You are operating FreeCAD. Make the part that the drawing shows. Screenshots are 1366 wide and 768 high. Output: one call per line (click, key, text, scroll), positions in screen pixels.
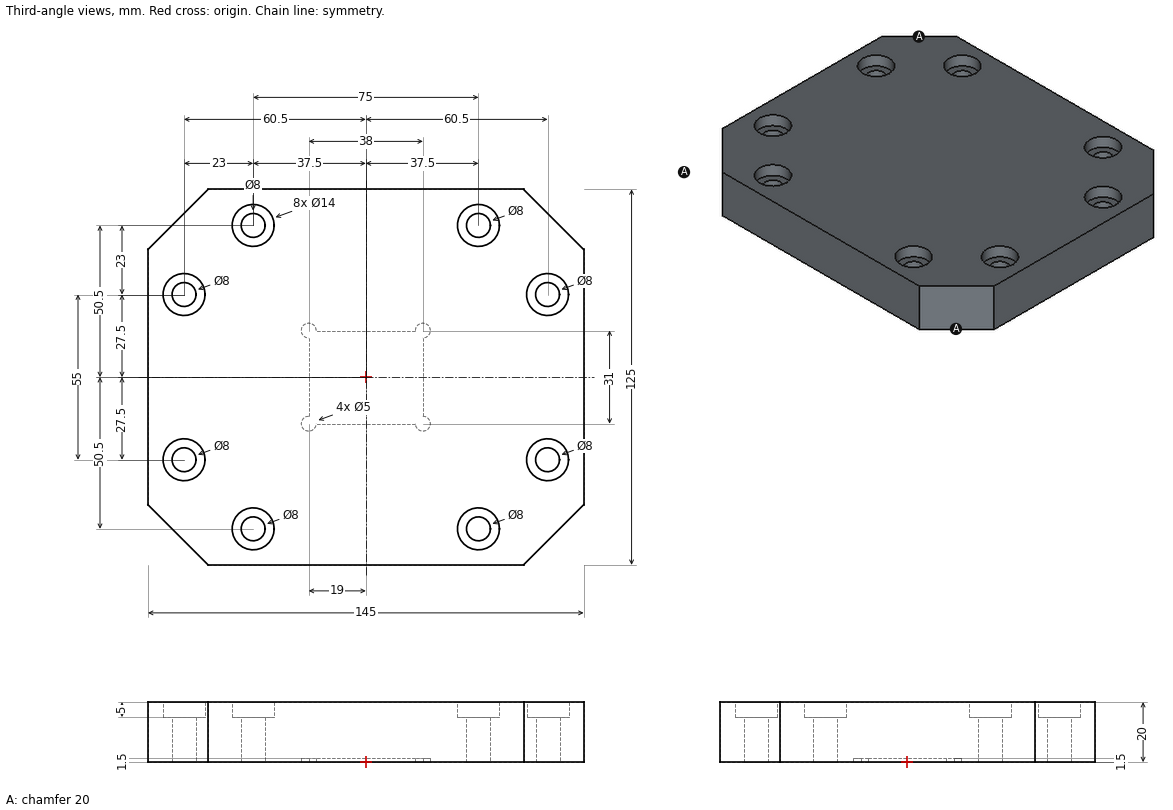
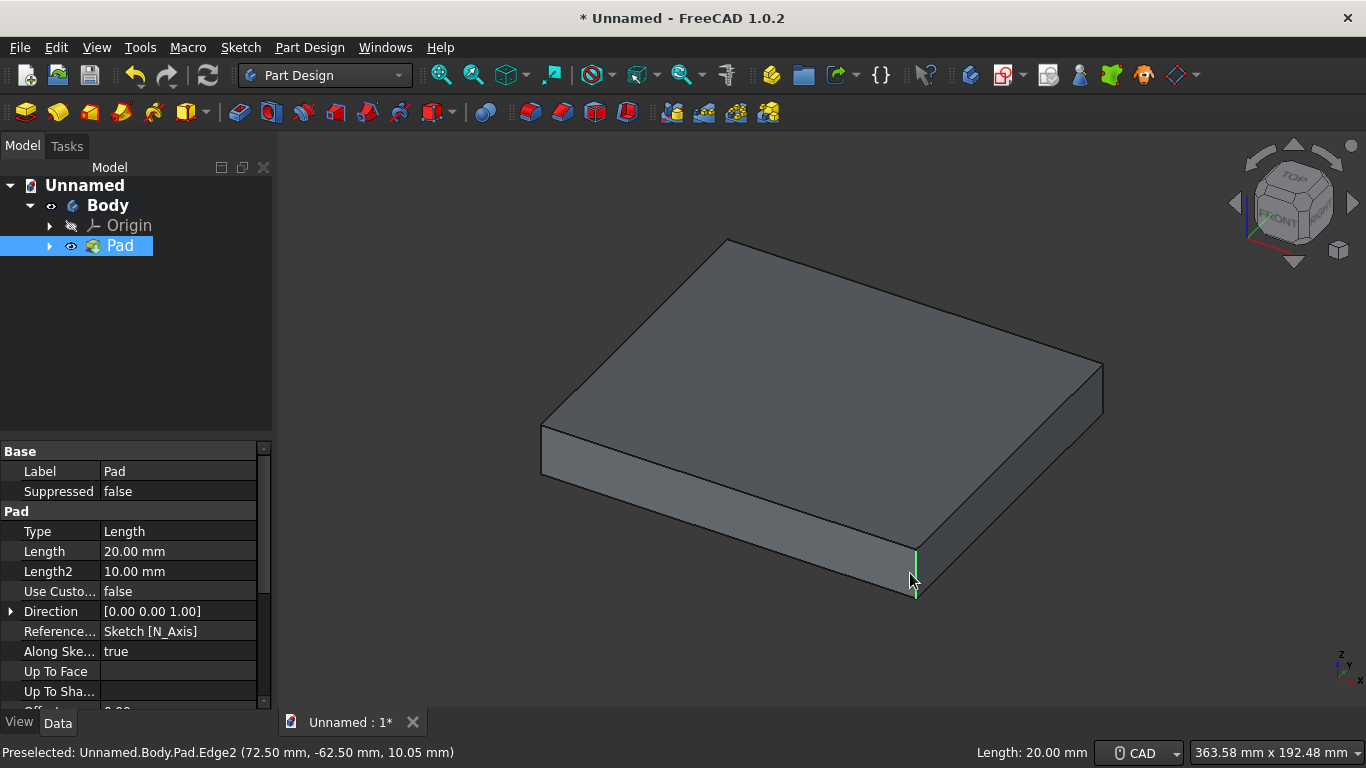
key(0)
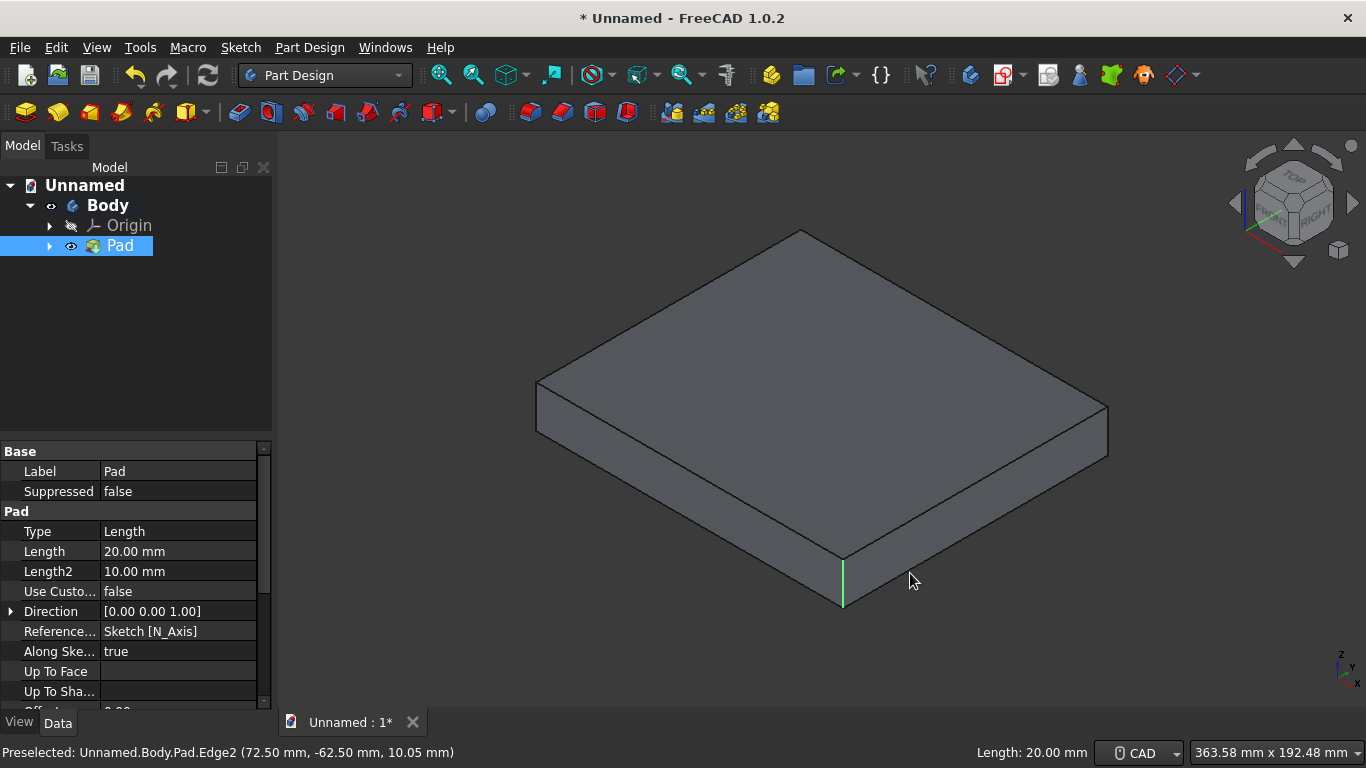
key(2)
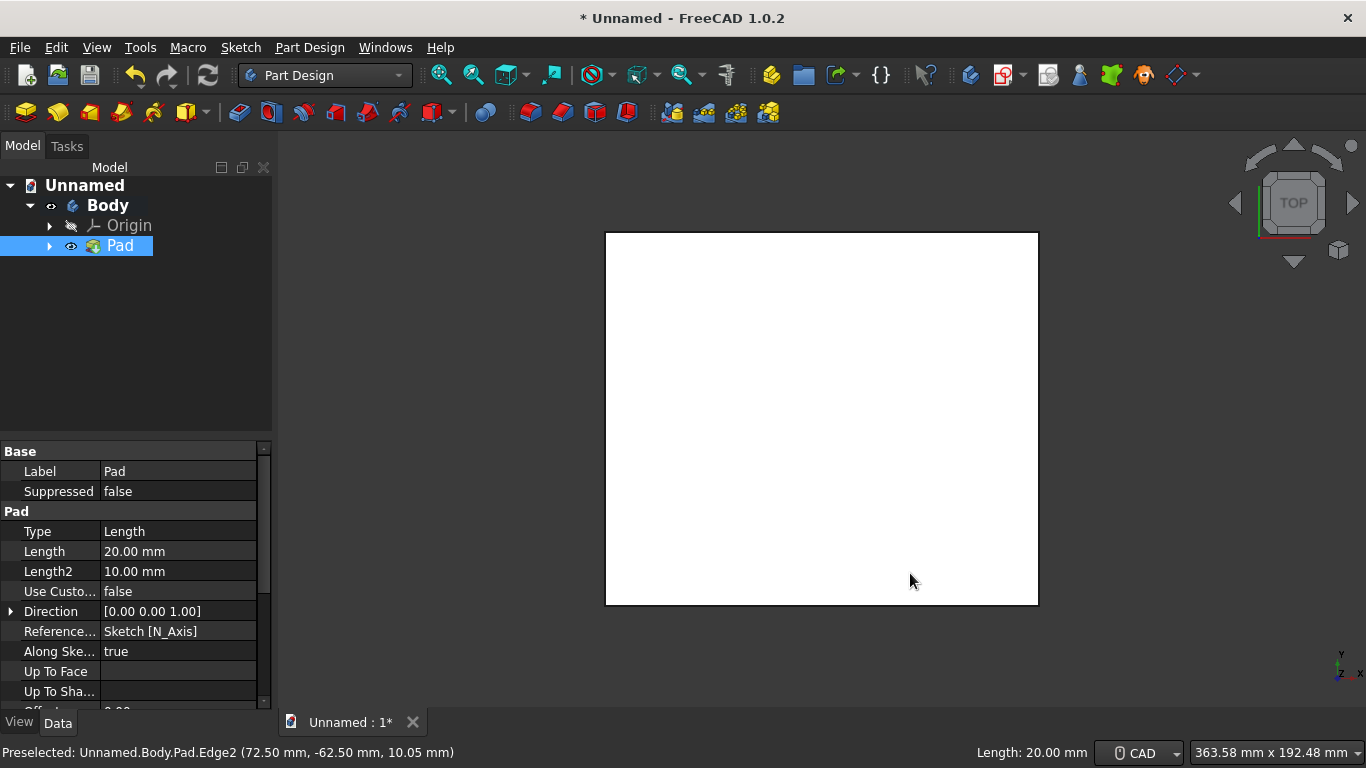
key(1)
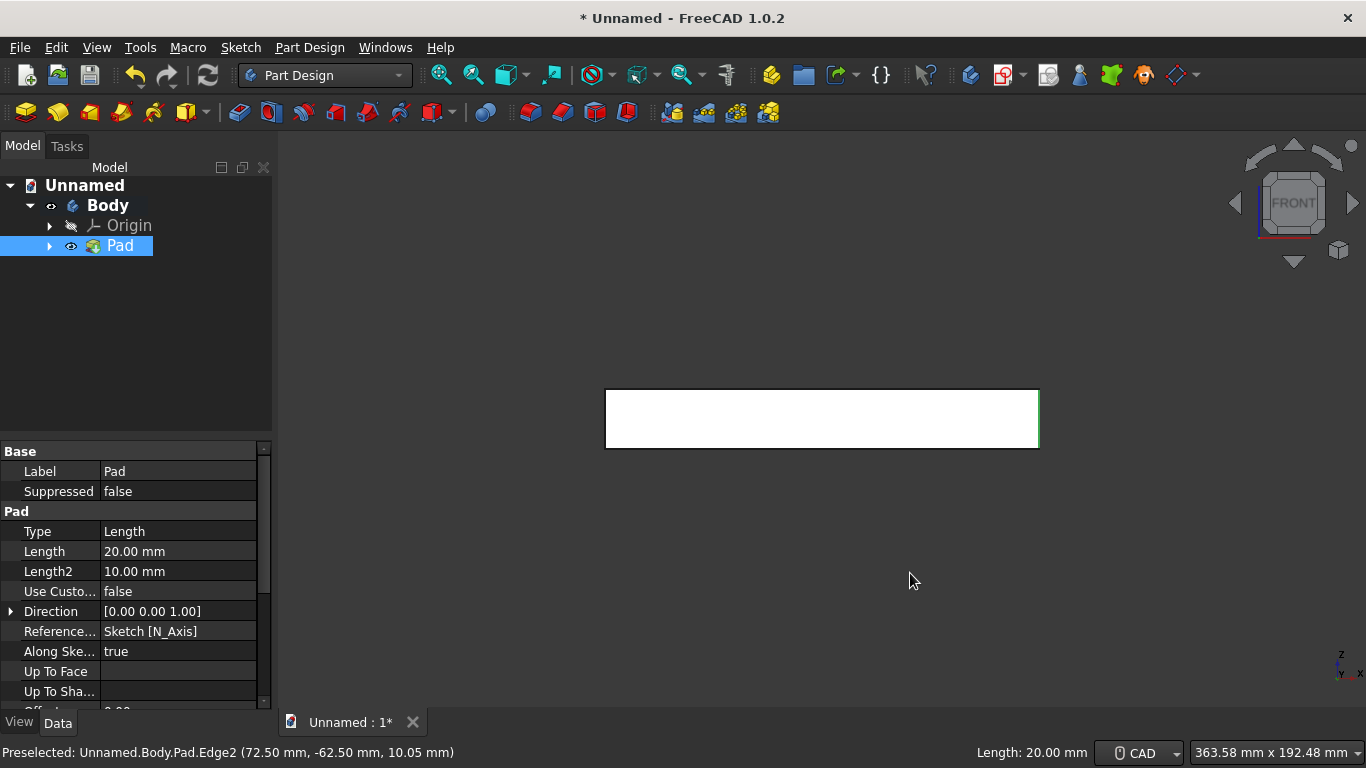
key(v)
key(f)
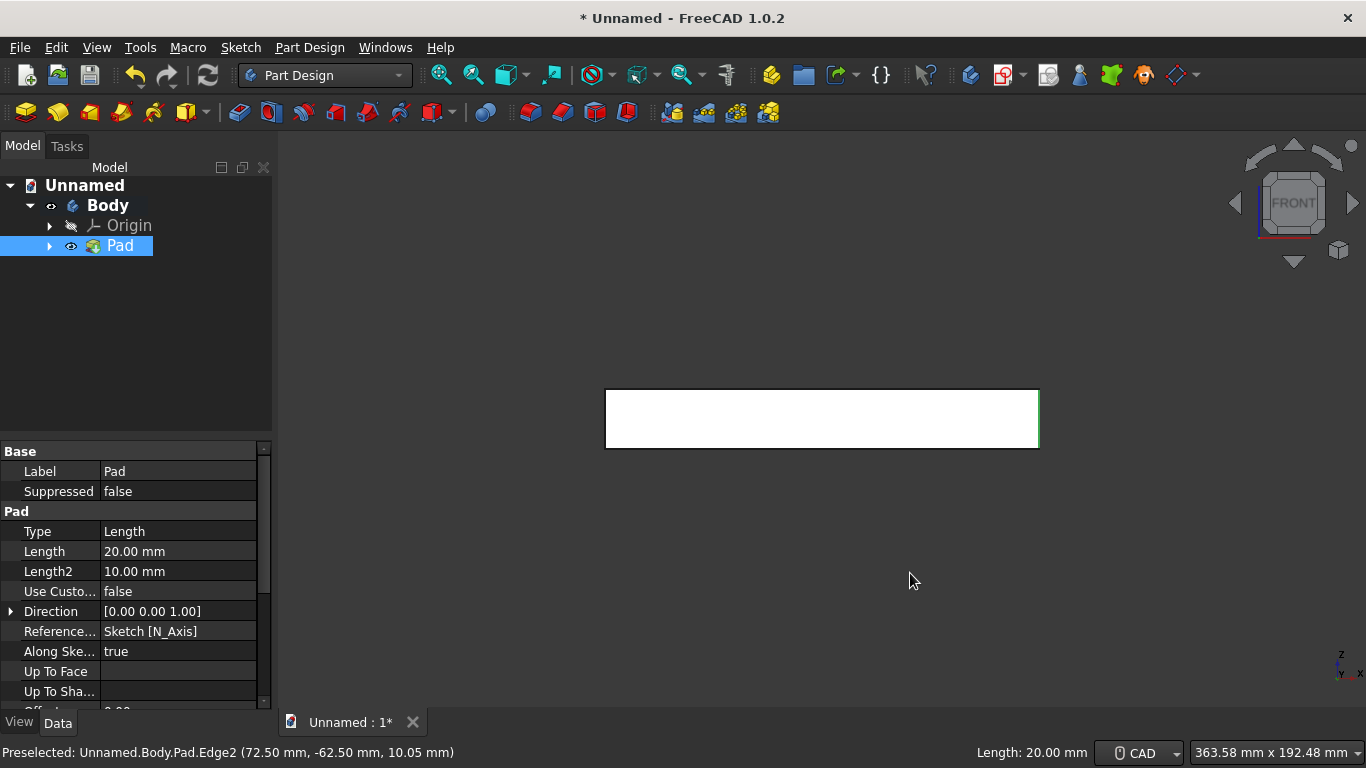
click(605, 418, ctrl)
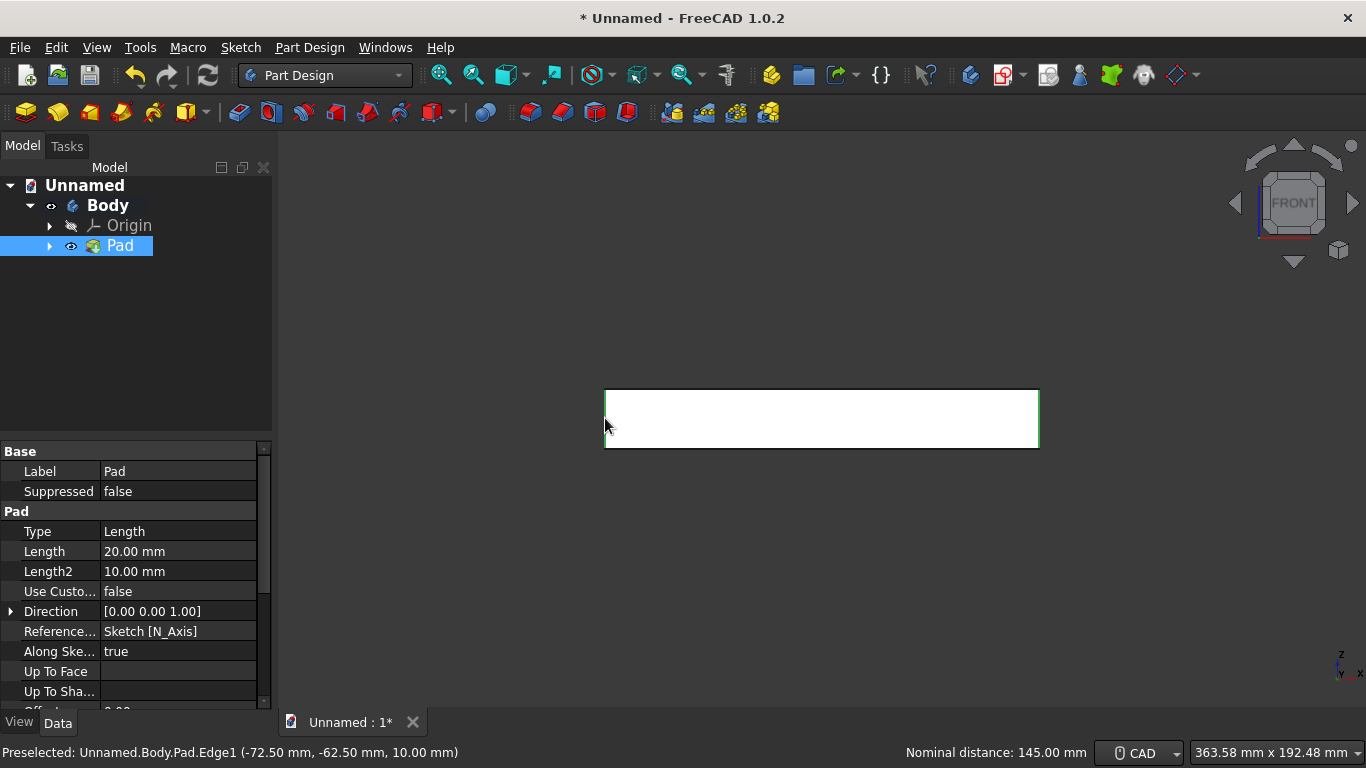
key(3)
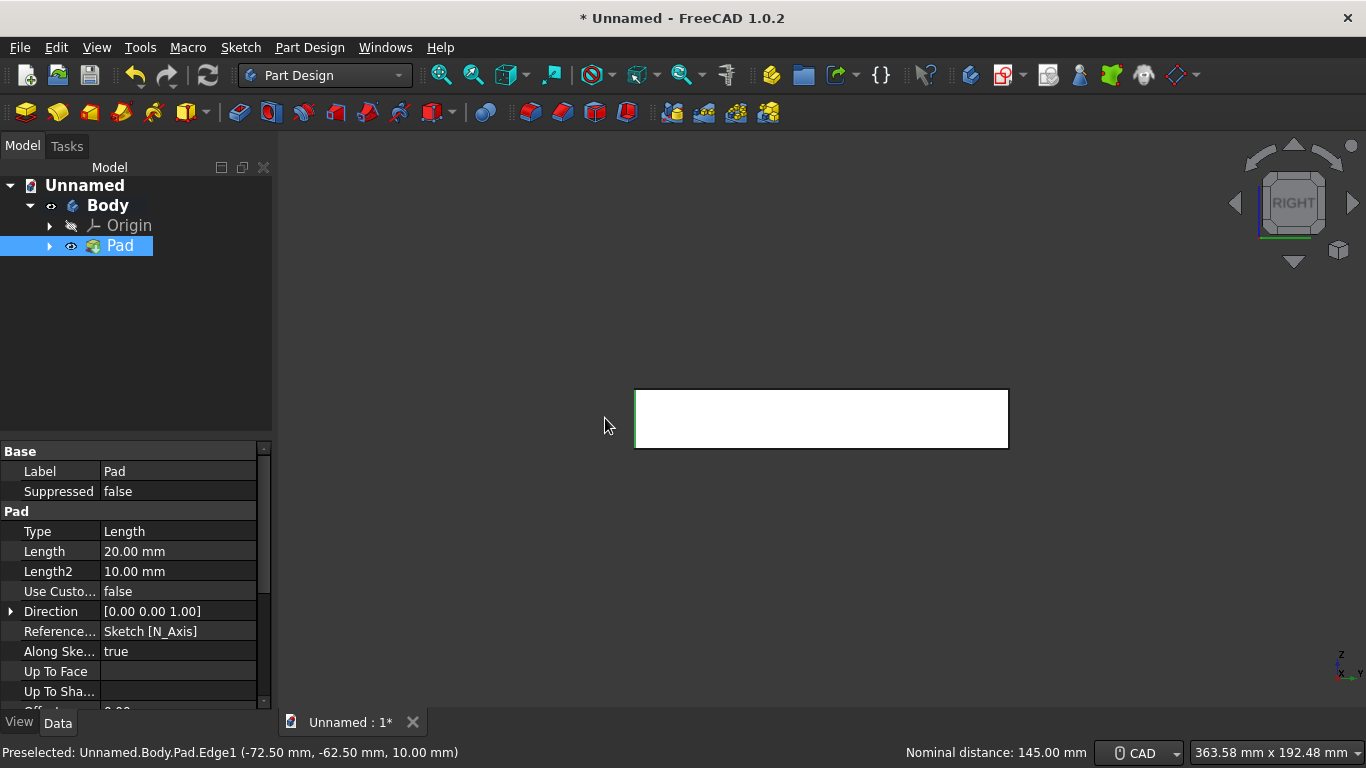
key(v)
key(f)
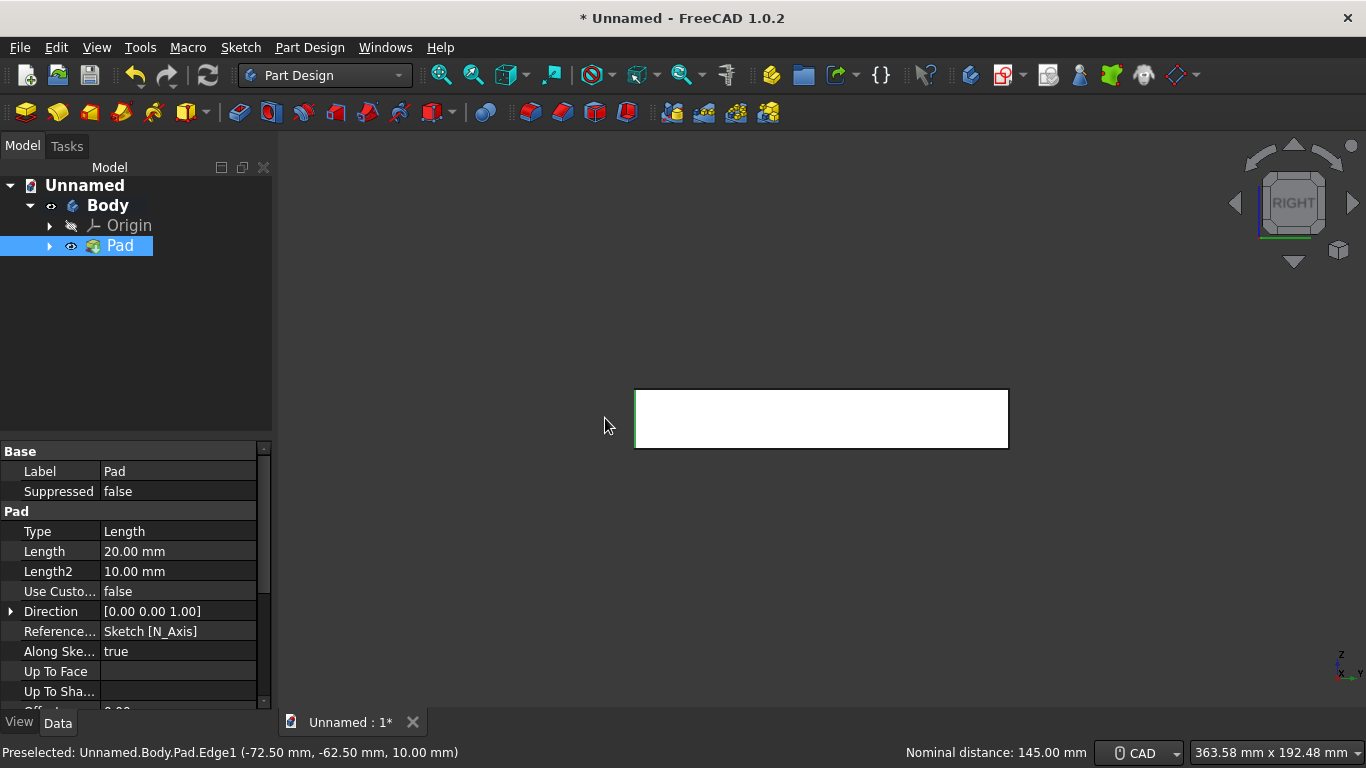
click(1009, 418, ctrl)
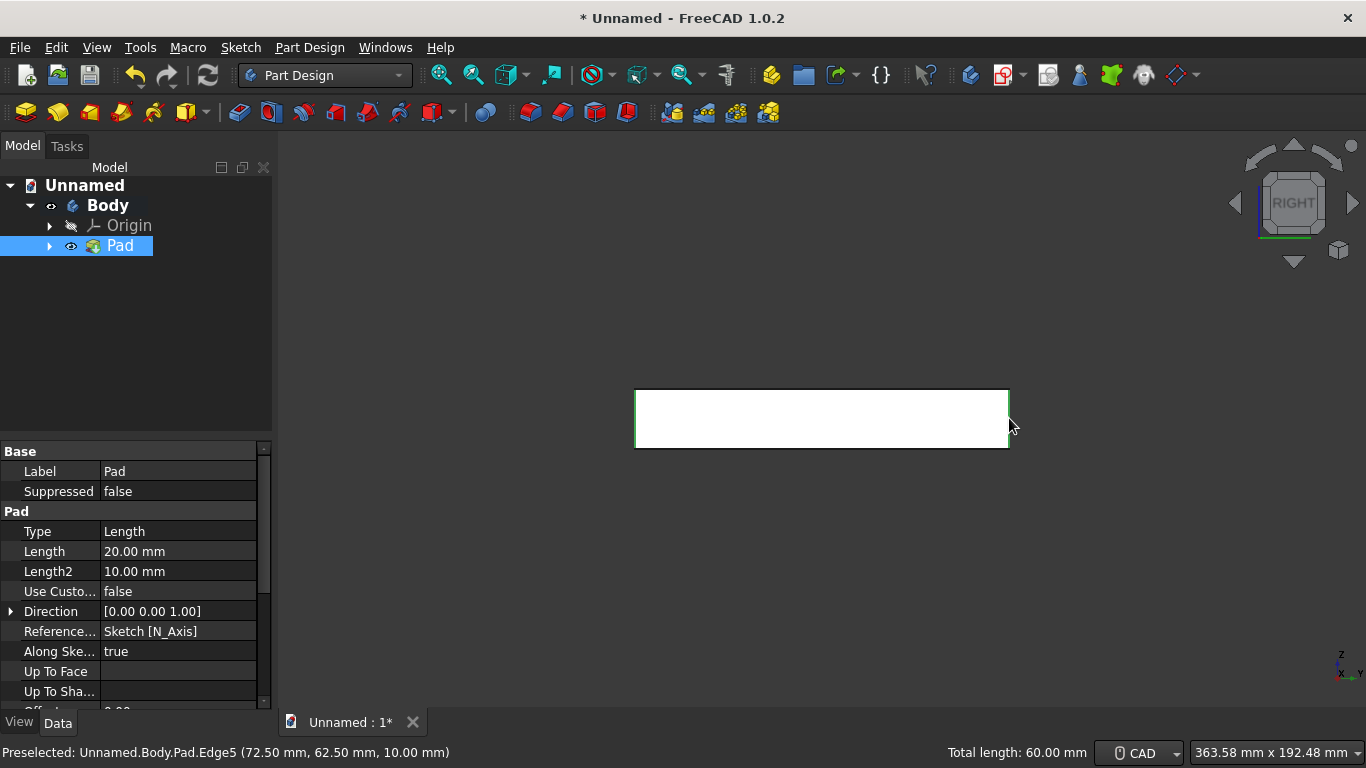
key(5)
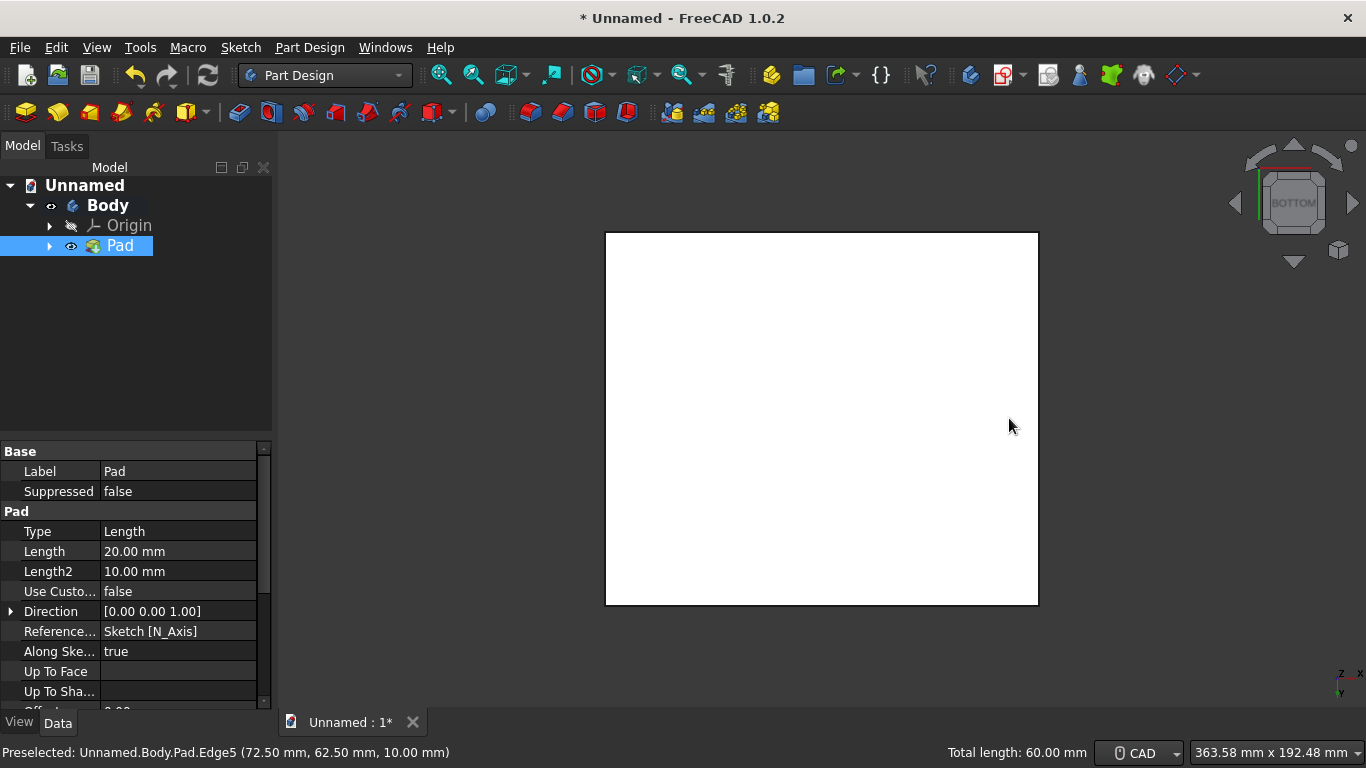
key(4)